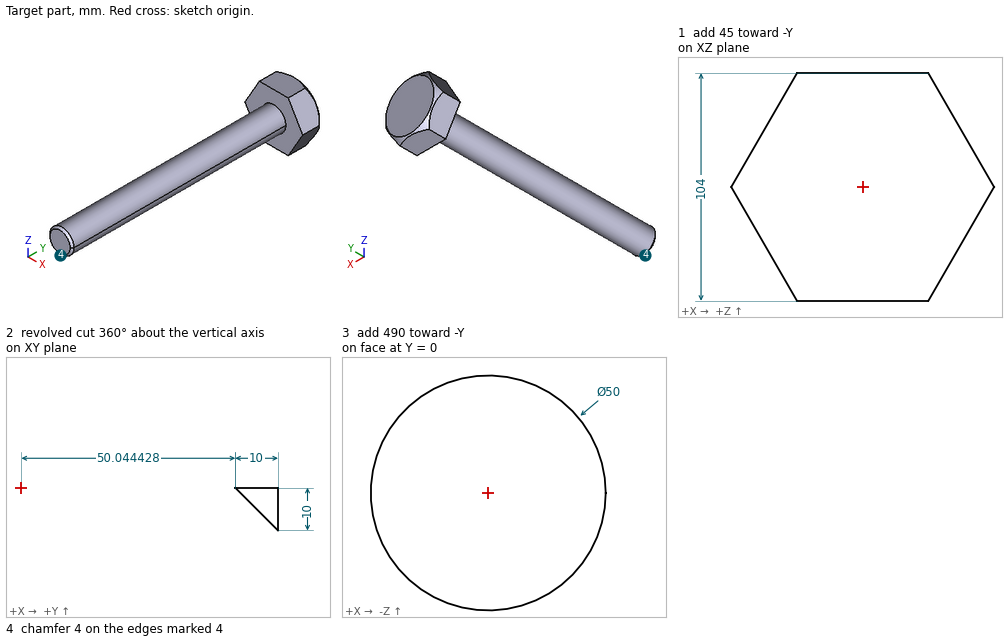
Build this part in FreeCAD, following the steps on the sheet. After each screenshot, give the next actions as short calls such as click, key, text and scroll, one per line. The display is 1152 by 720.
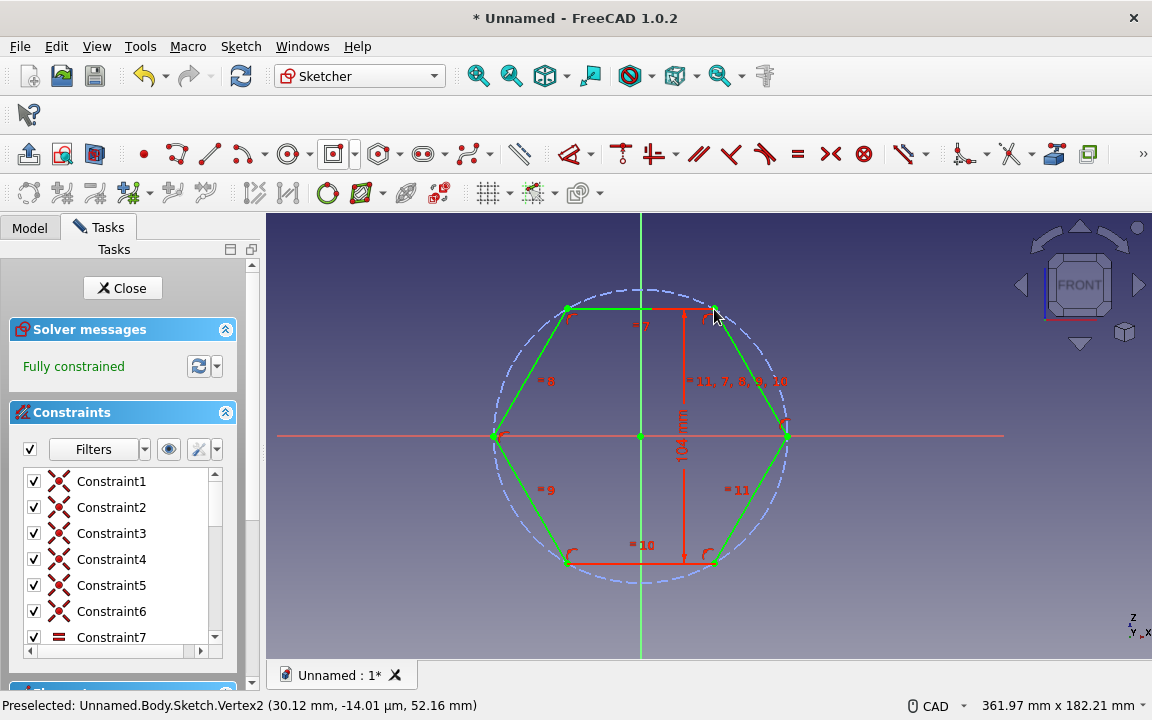
click(123, 288)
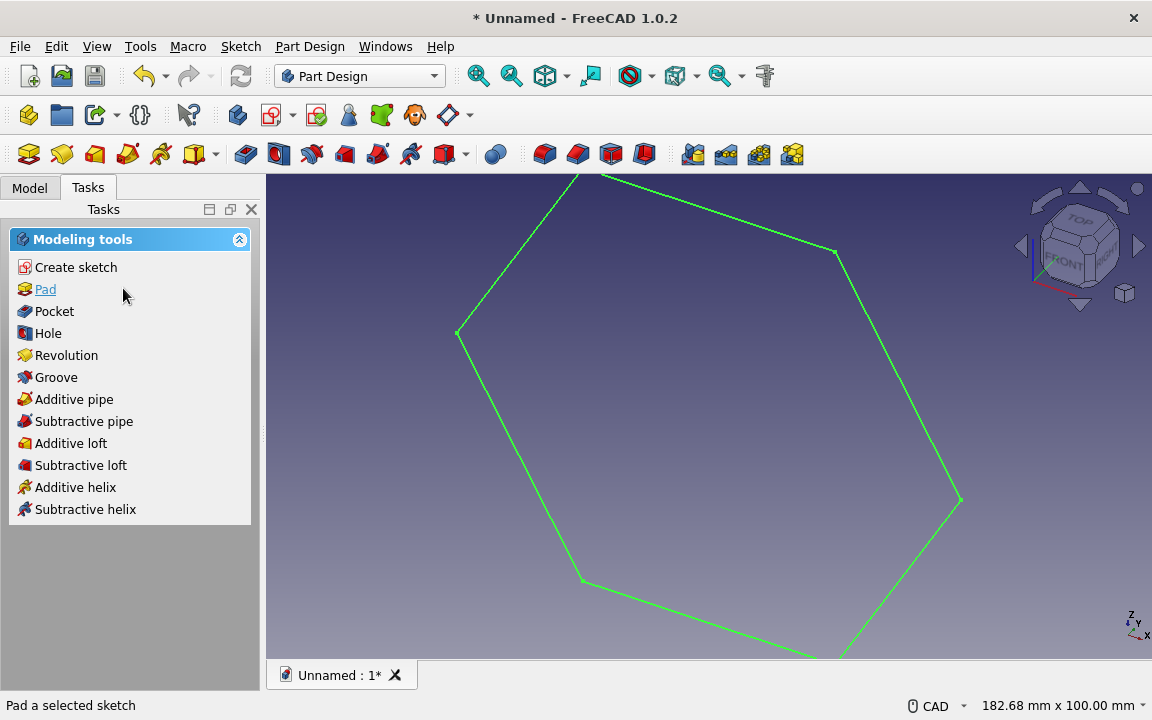
click(29, 154)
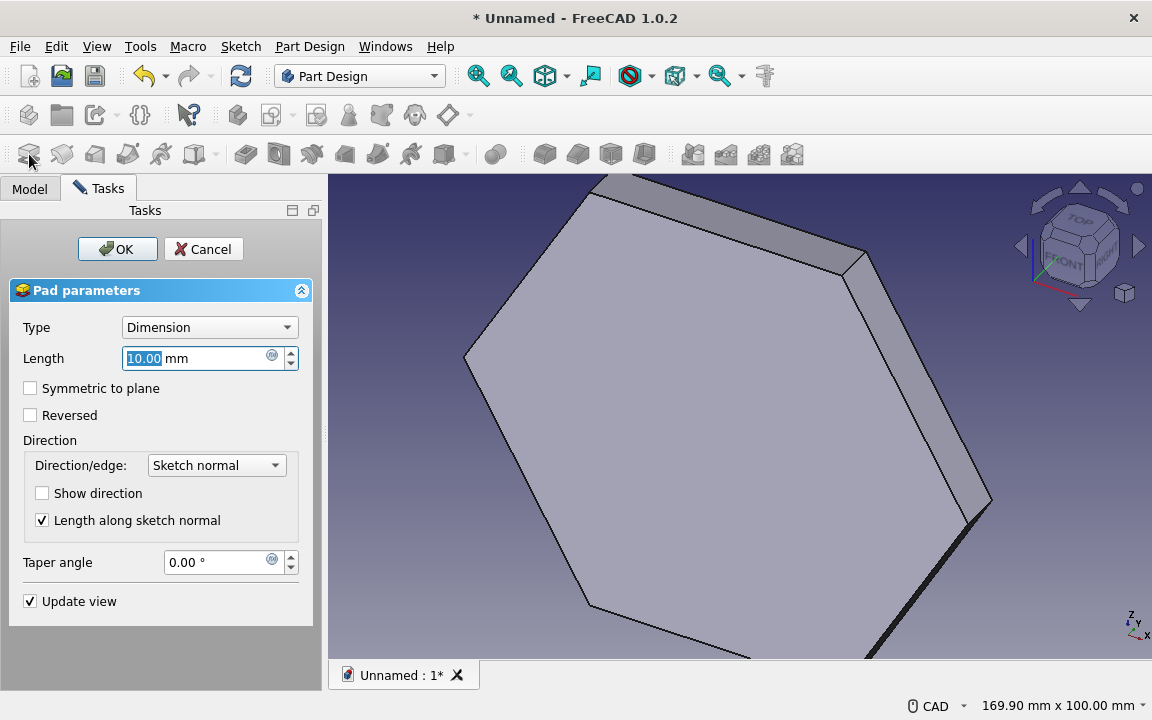
text(45)
key(Tab)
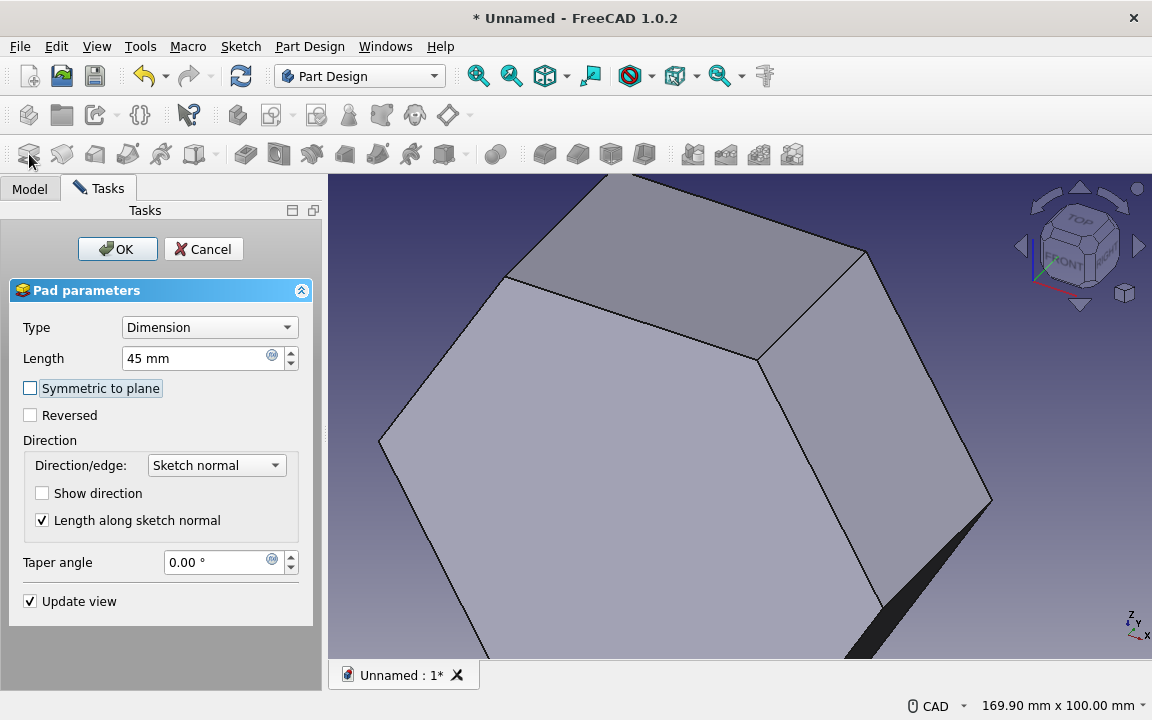
click(118, 249)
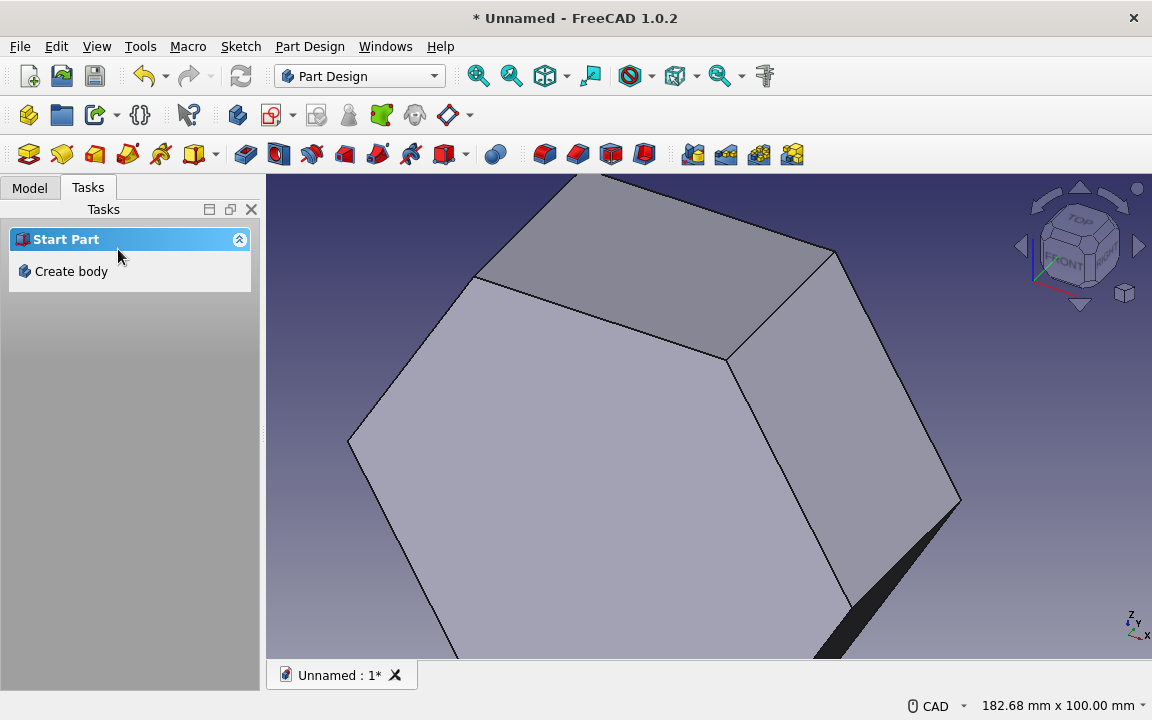
click(479, 76)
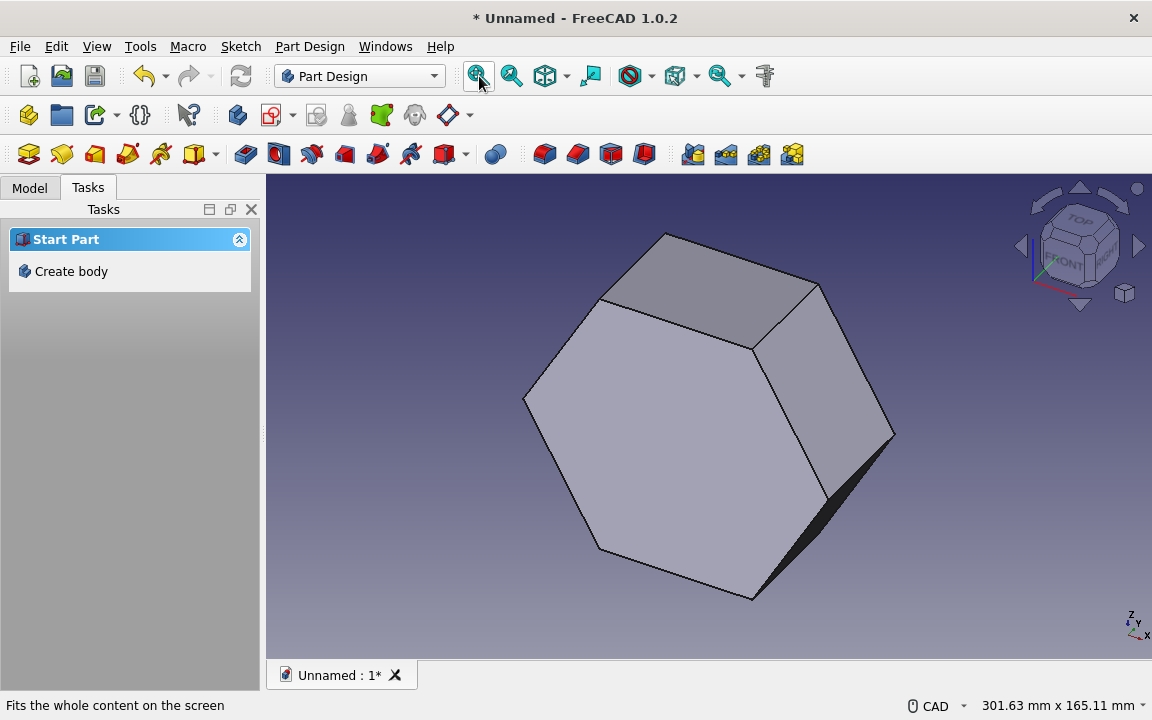
click(270, 116)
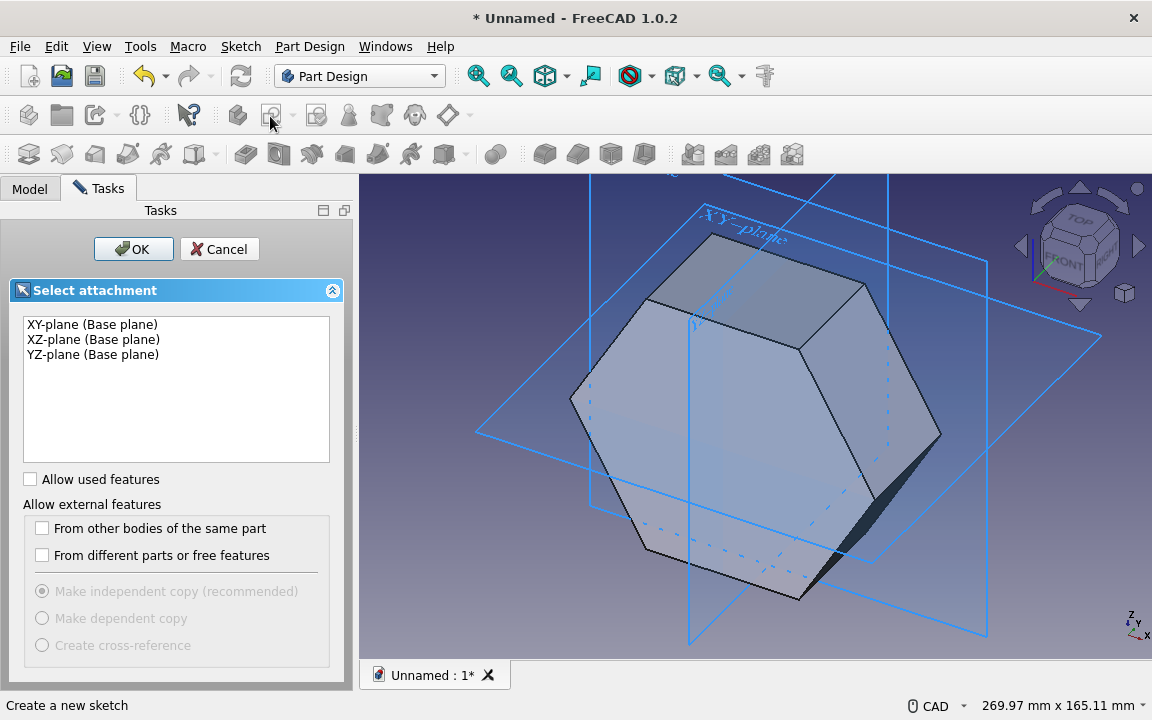
click(84, 324)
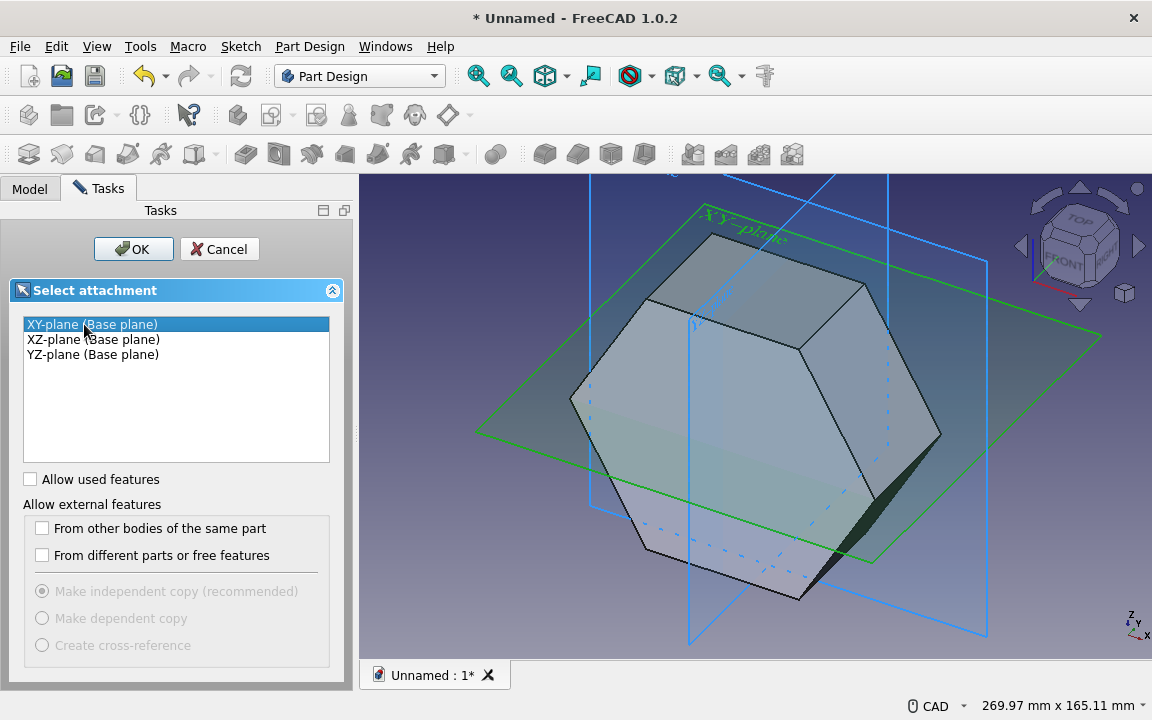
click(134, 249)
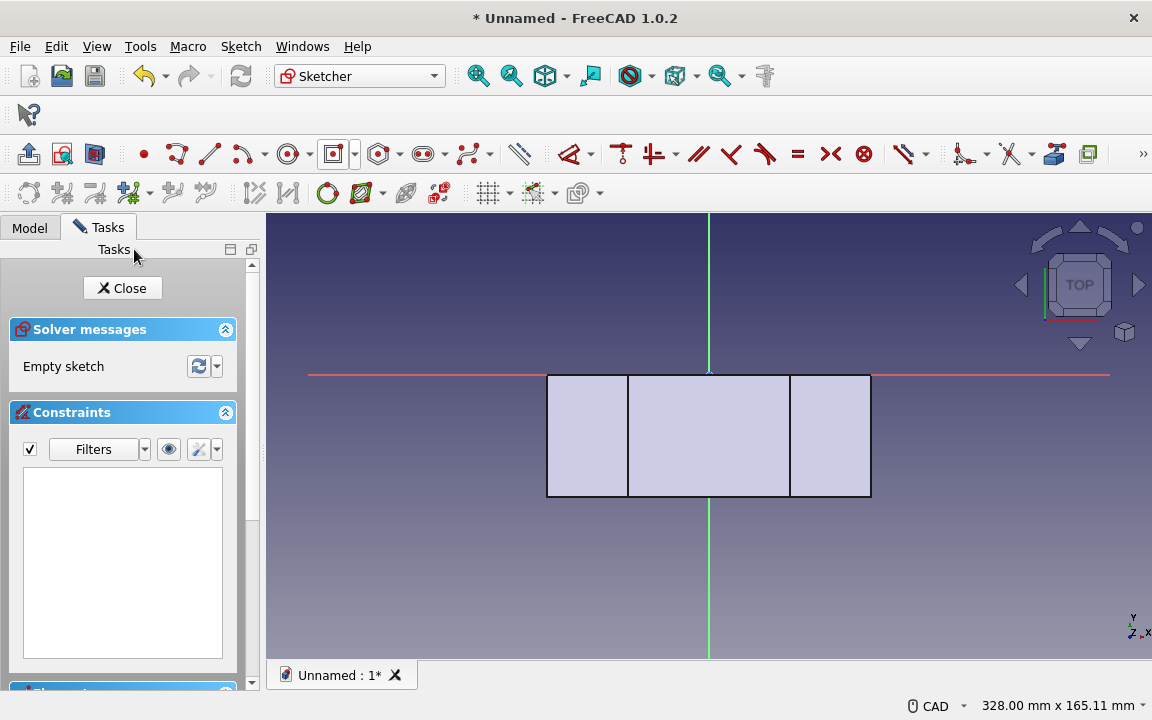
click(95, 154)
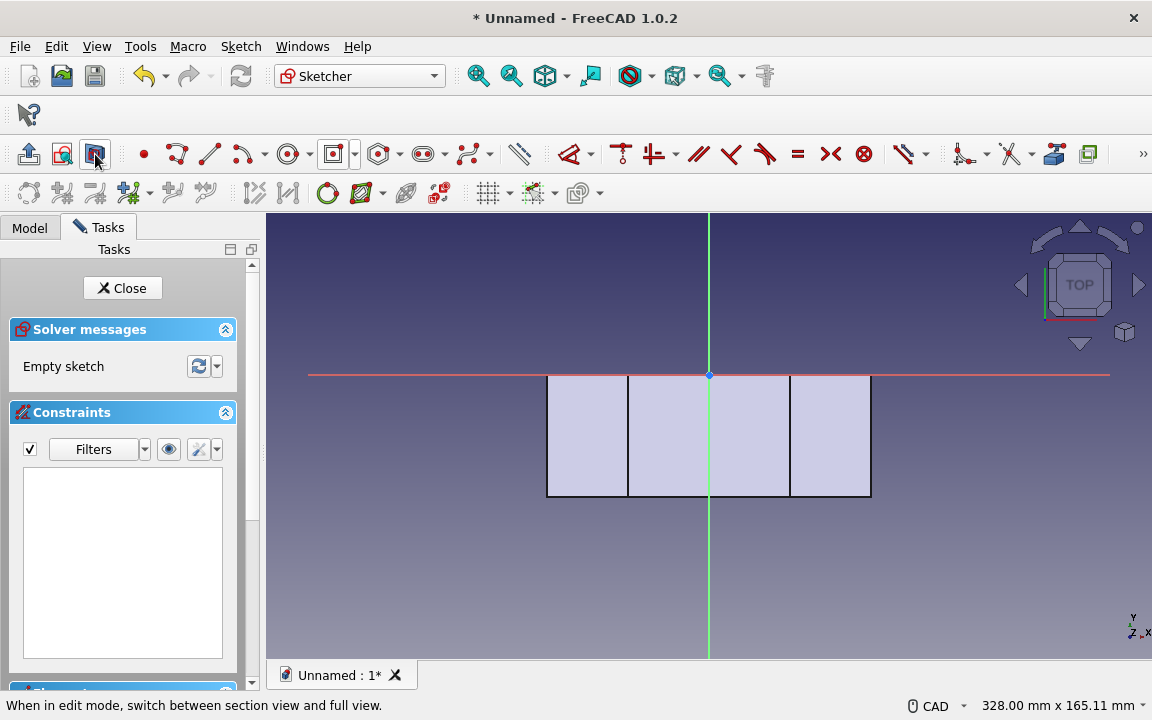
scroll(879, 384, up, 12)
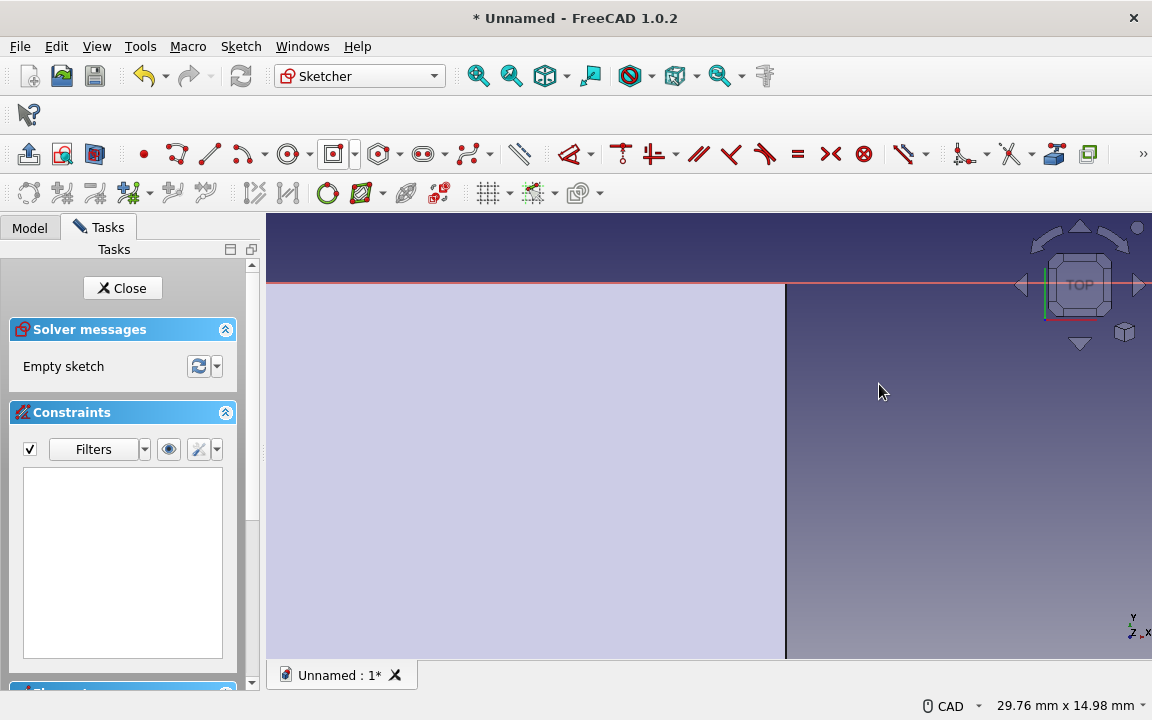
click(177, 154)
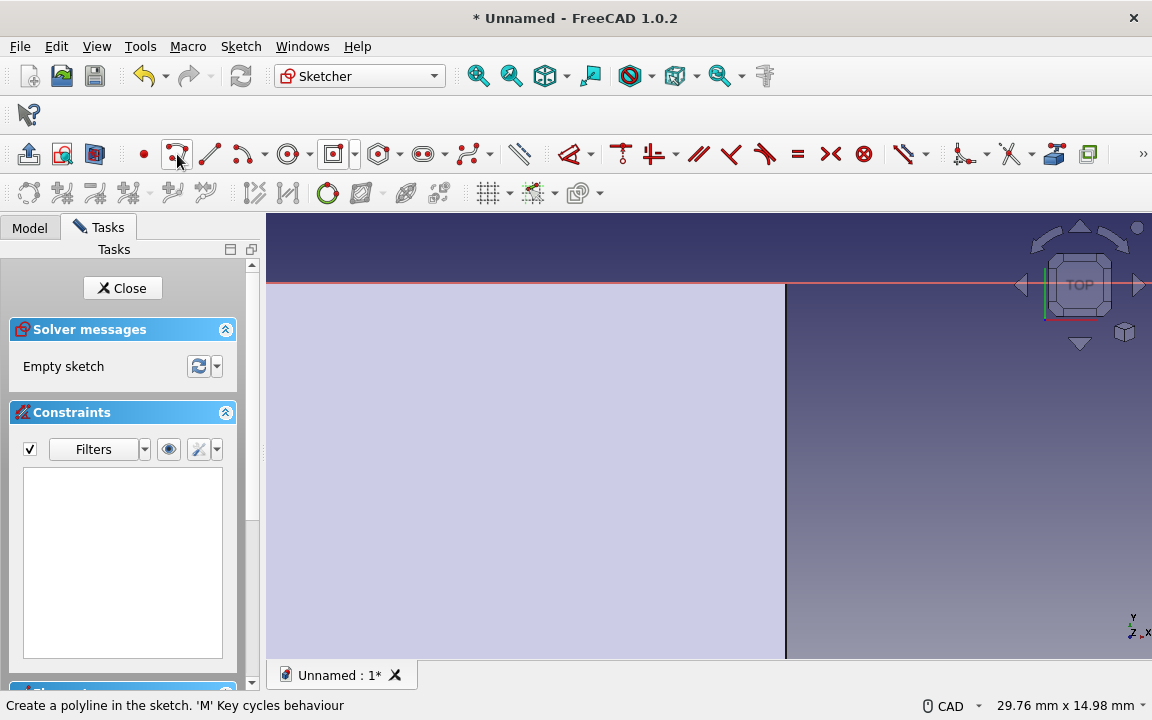
click(488, 283)
click(786, 581)
click(786, 292)
click(488, 283)
key(Escape)
key(Escape)